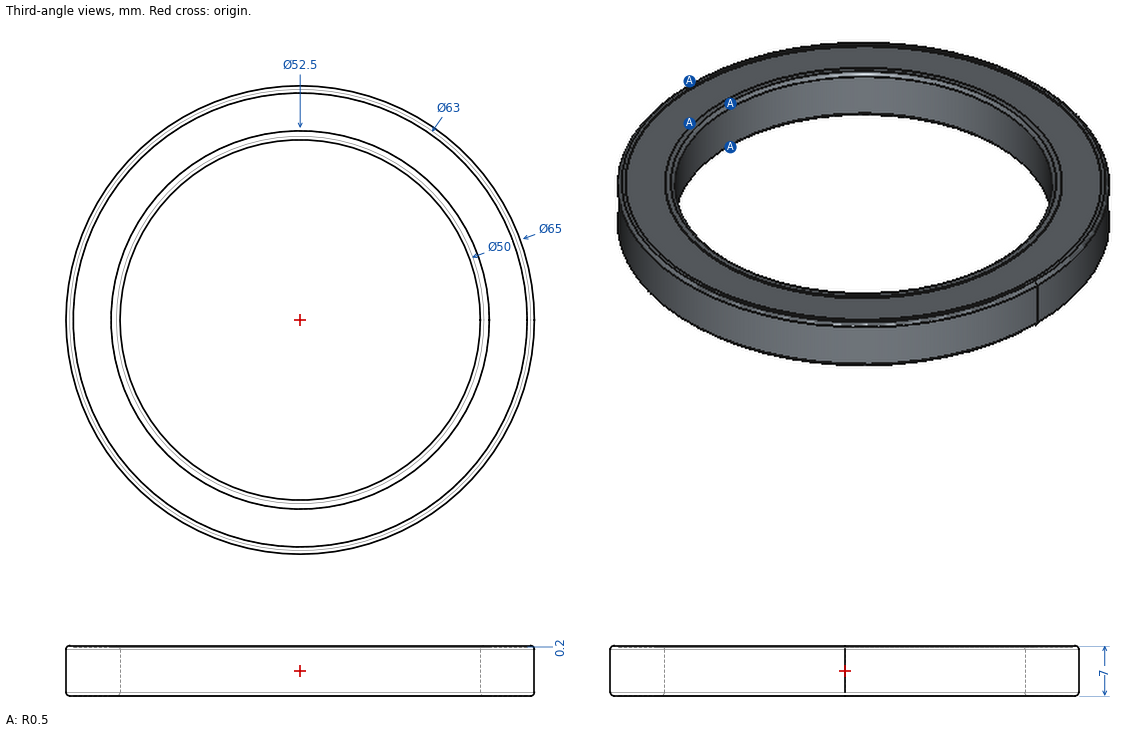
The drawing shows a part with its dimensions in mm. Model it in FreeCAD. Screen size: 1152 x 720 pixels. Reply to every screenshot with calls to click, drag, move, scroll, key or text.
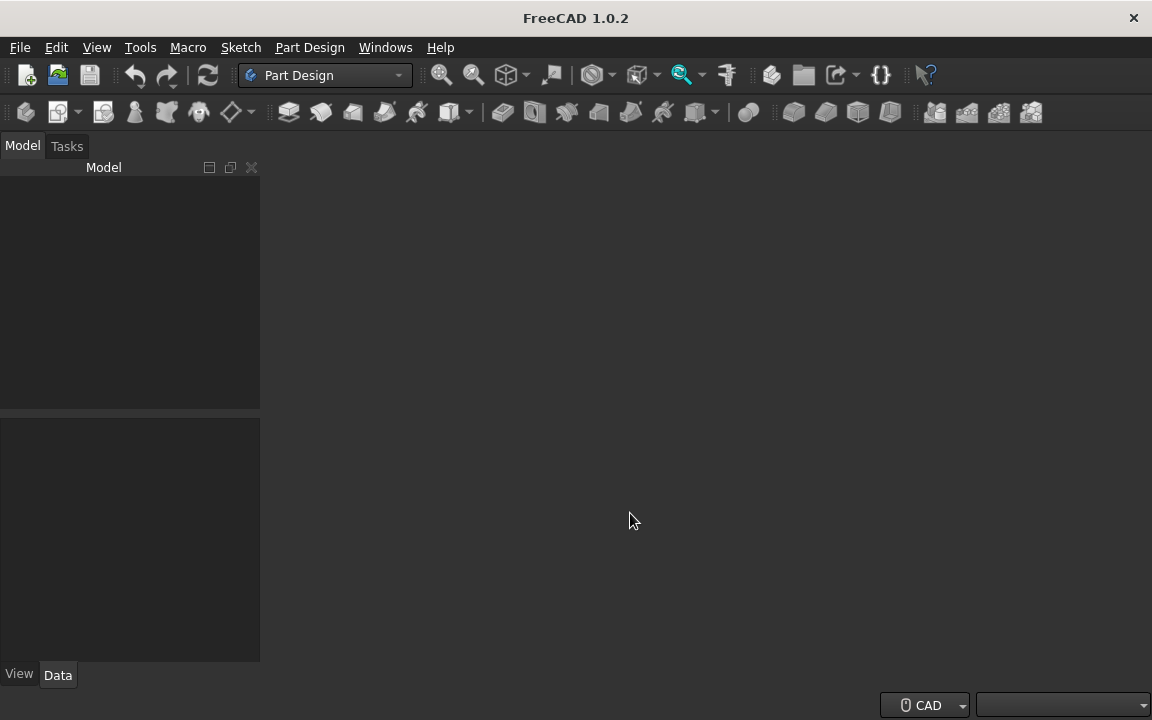
key(ctrl+n)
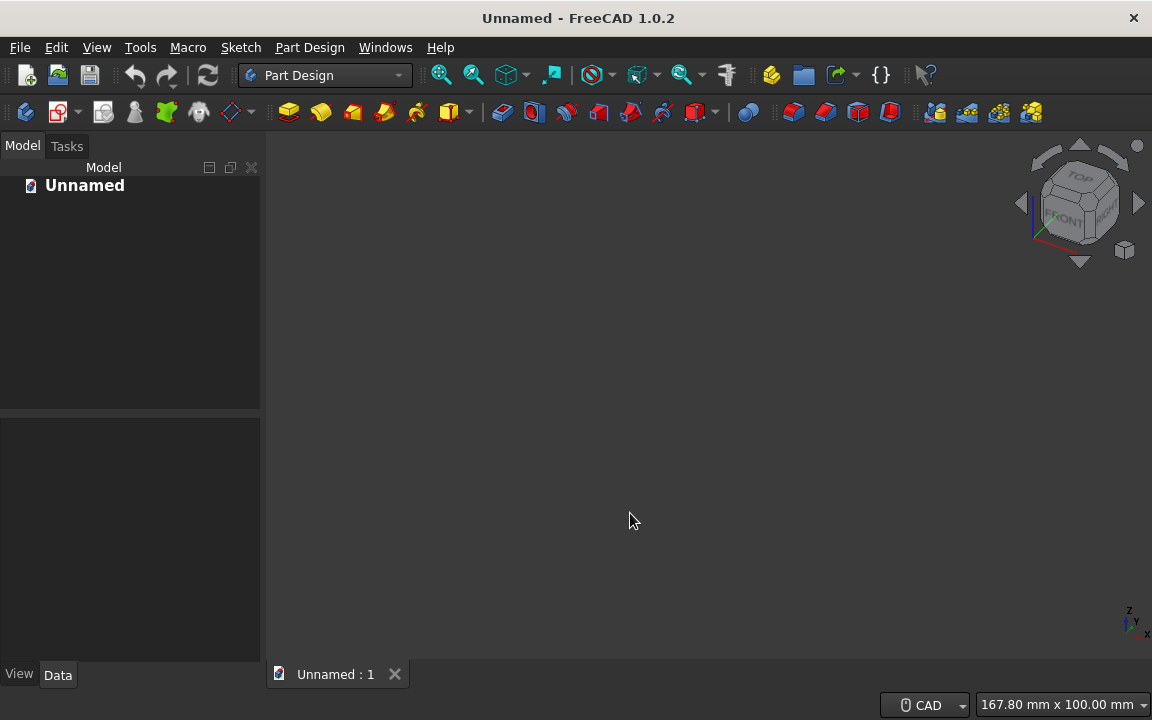
click(58, 112)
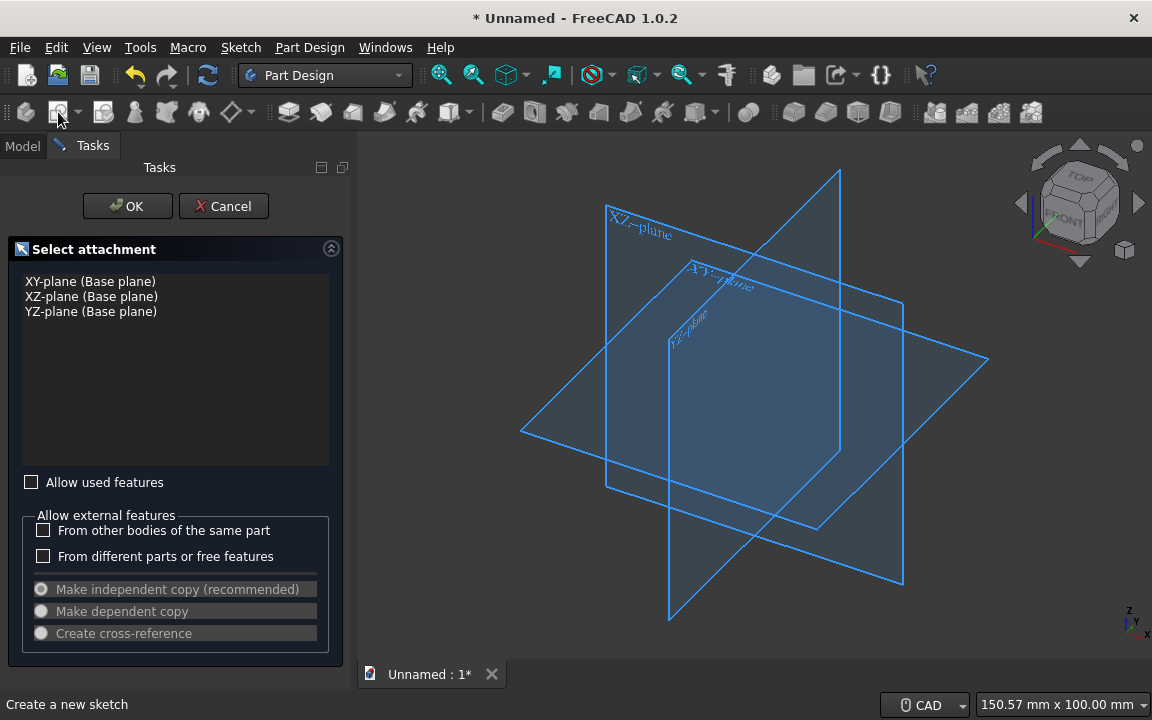
click(82, 282)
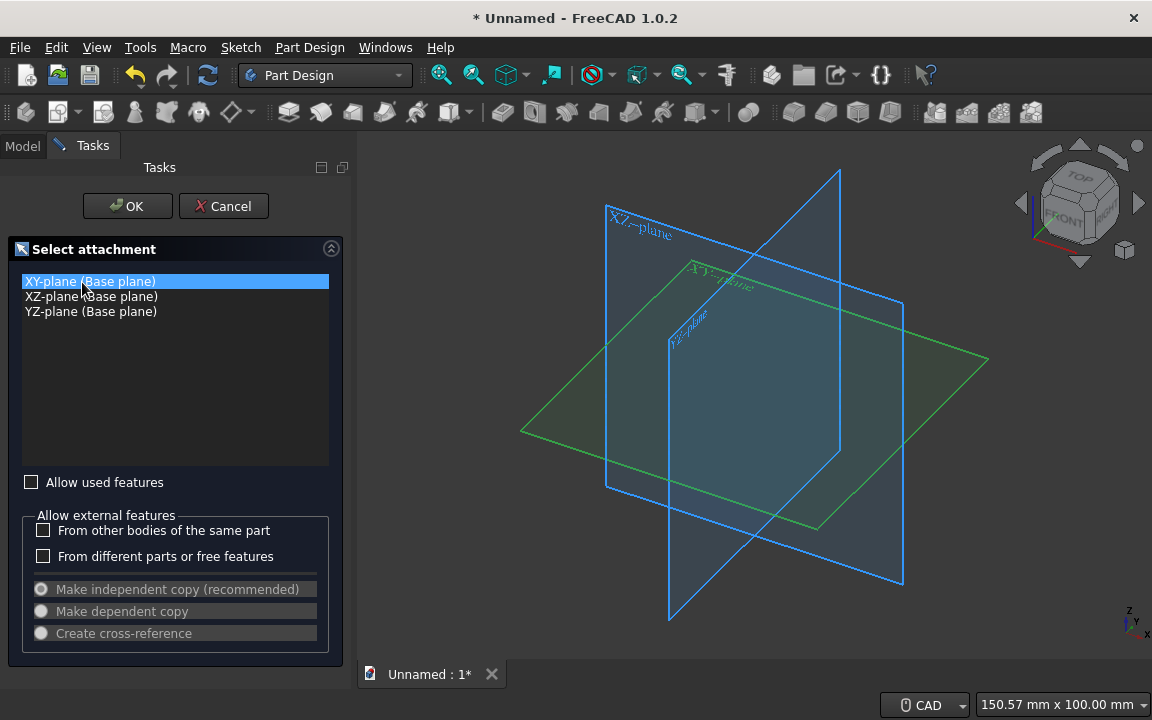
click(128, 206)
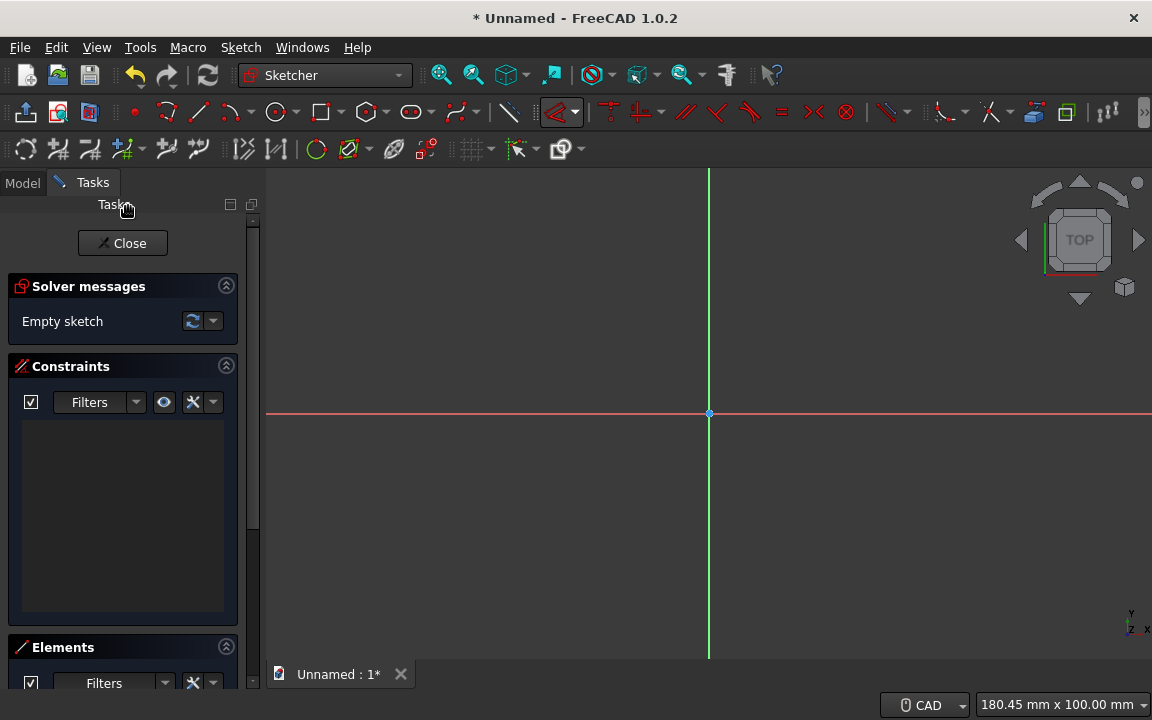
click(276, 112)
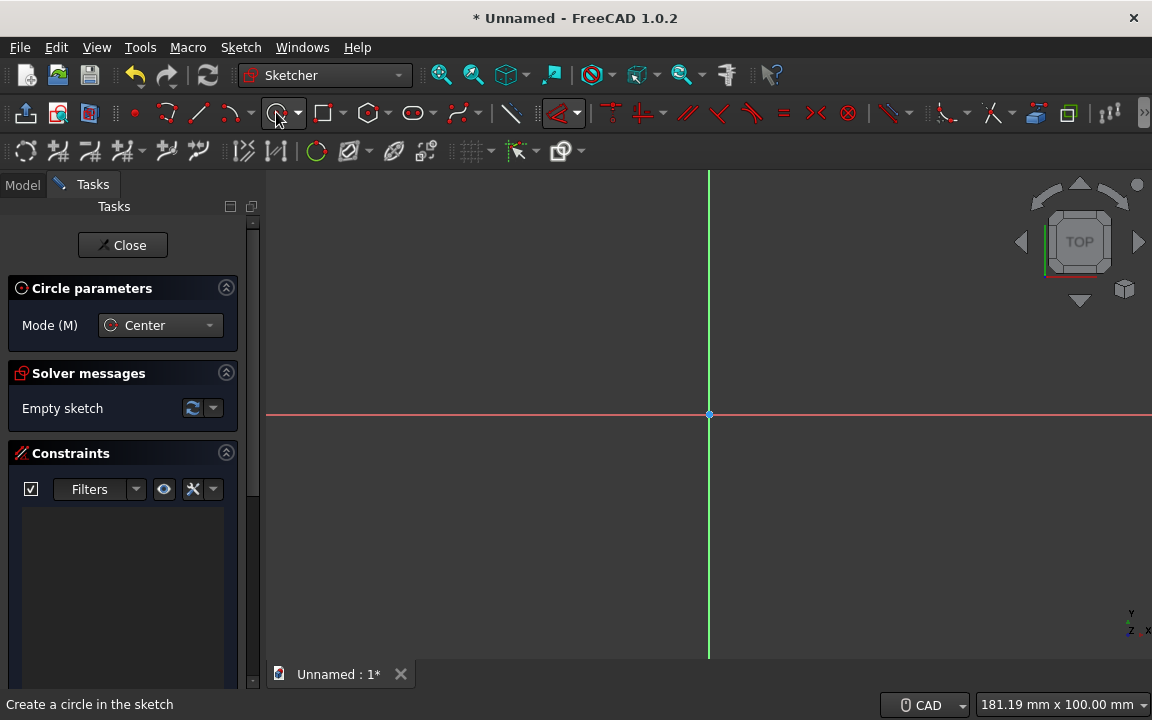
click(709, 414)
click(821, 302)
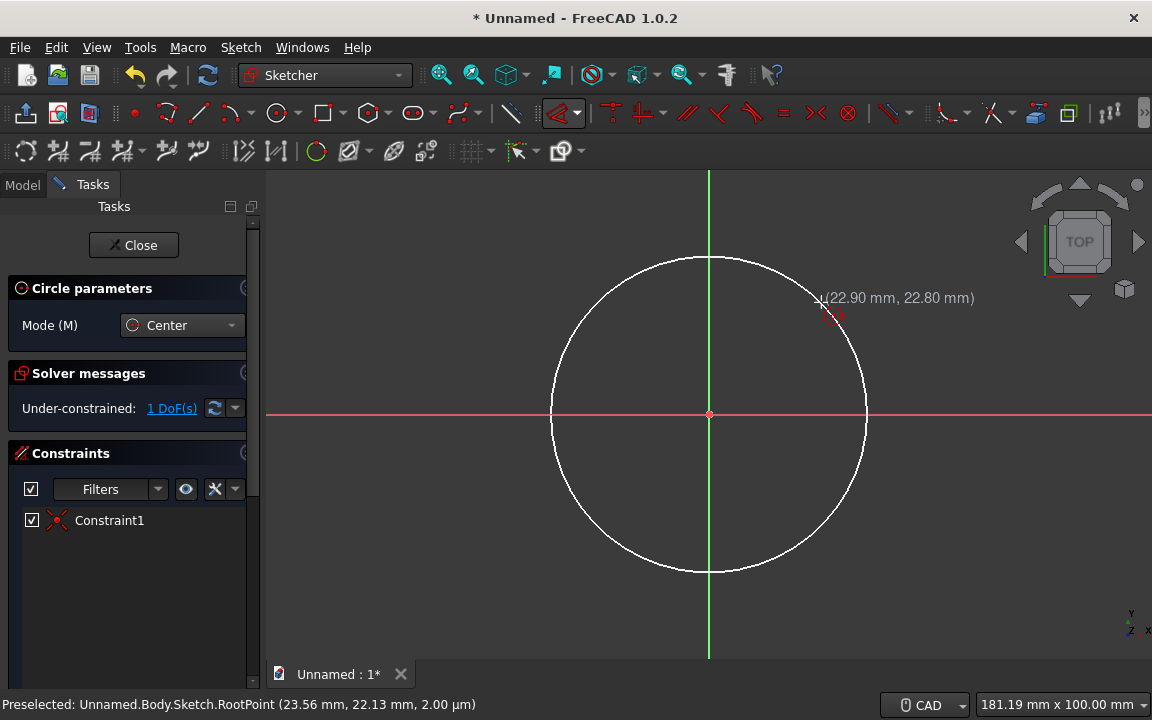
click(709, 414)
click(795, 328)
key(Escape)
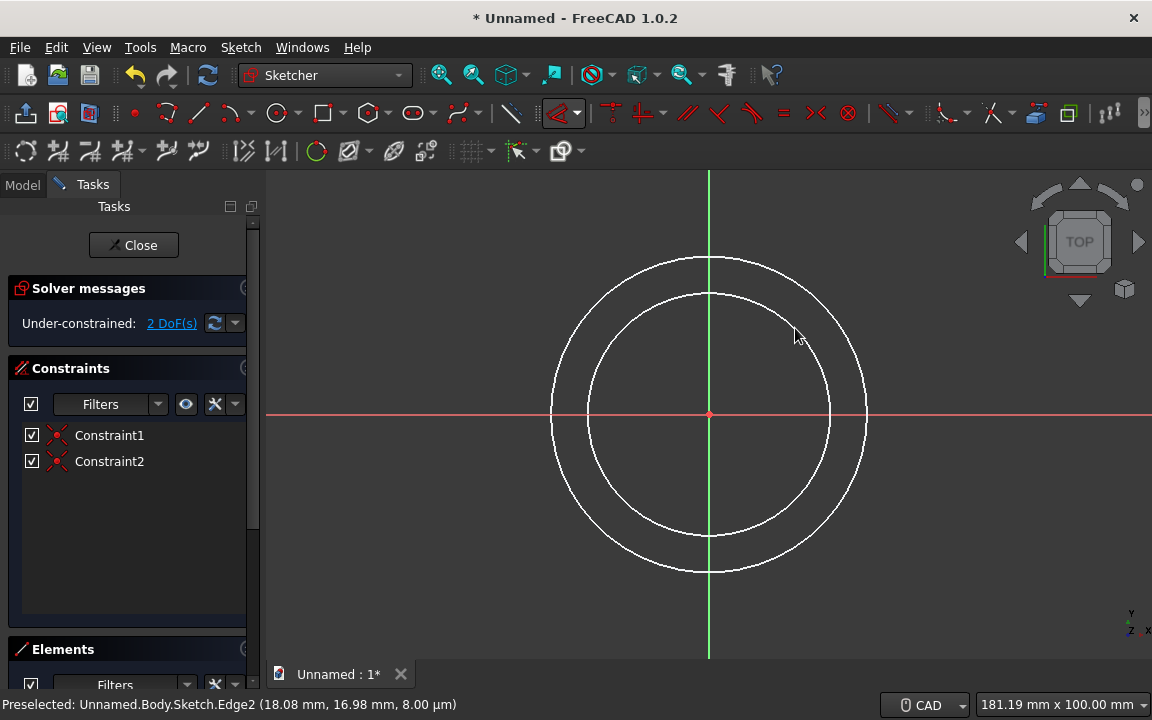
click(820, 302)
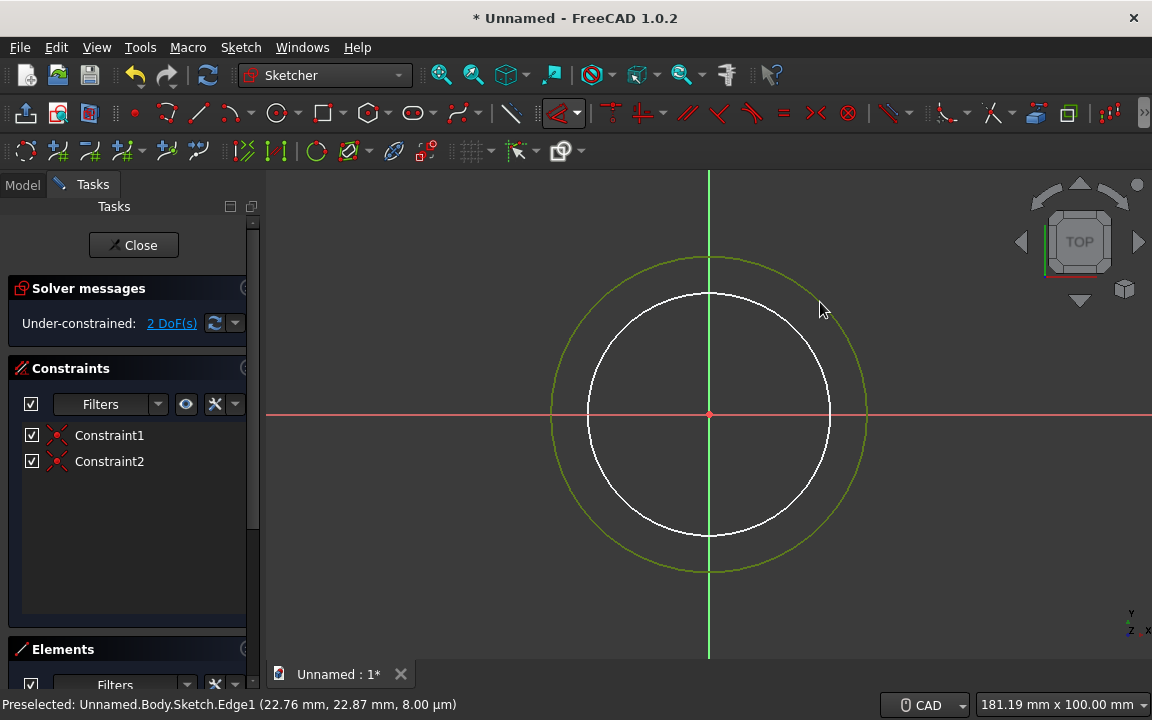
click(580, 114)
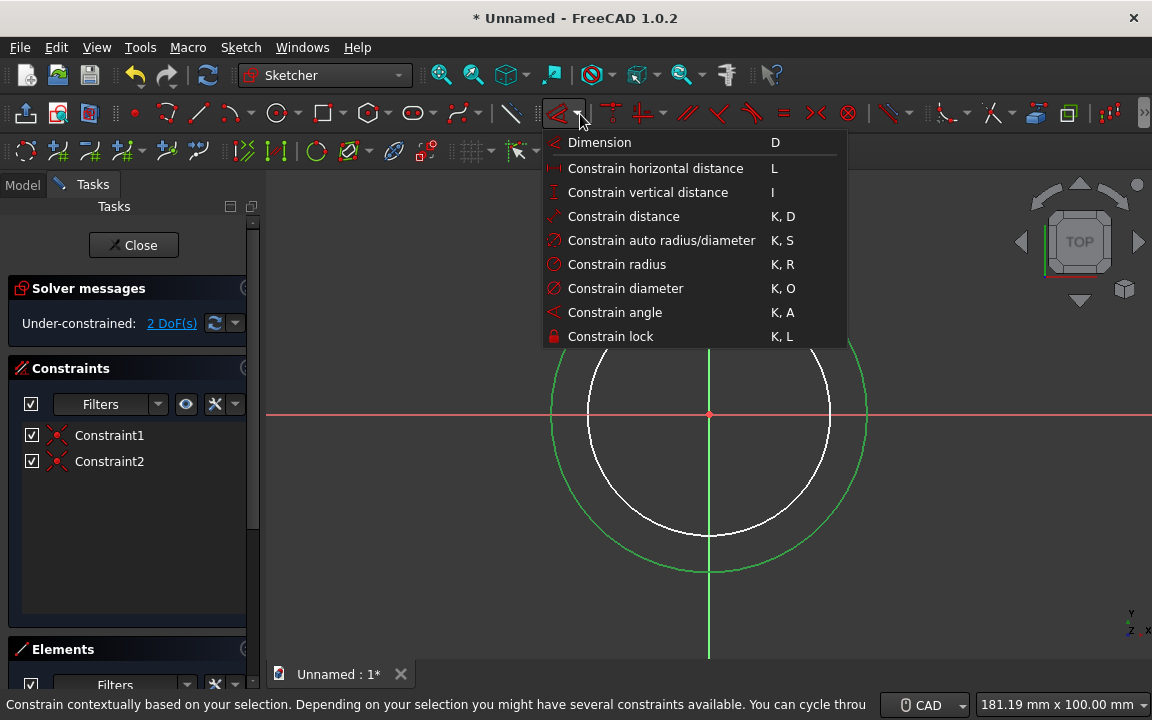
click(695, 288)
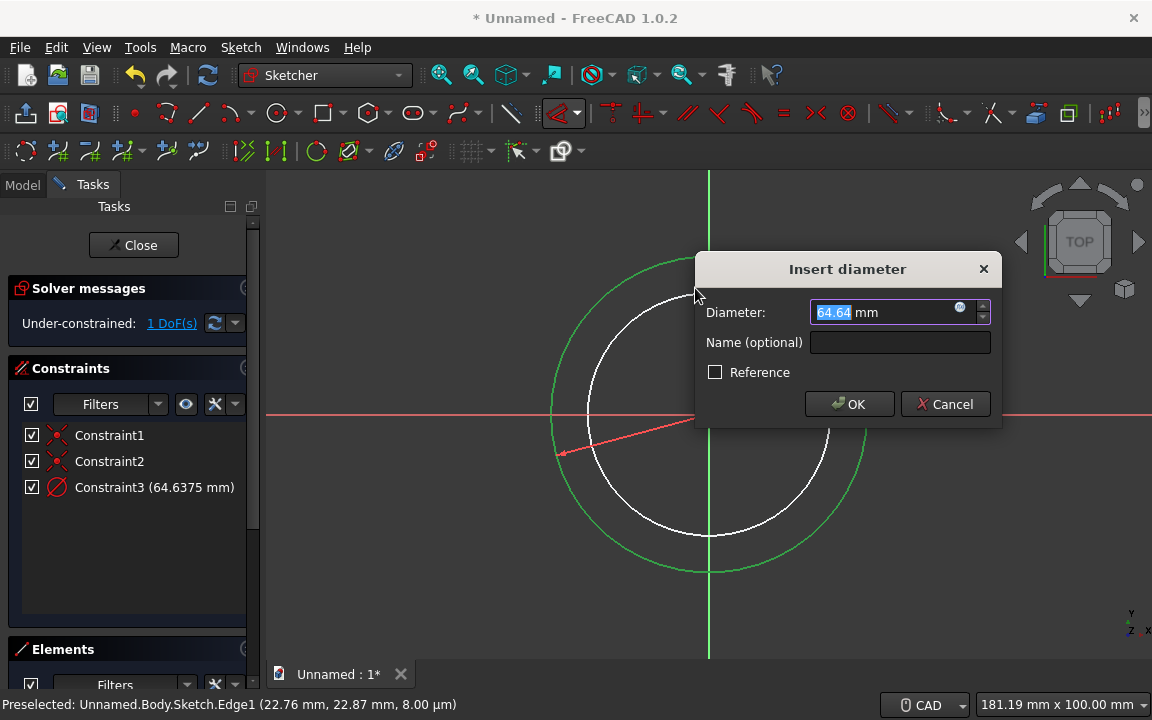
text(65)
key(Return)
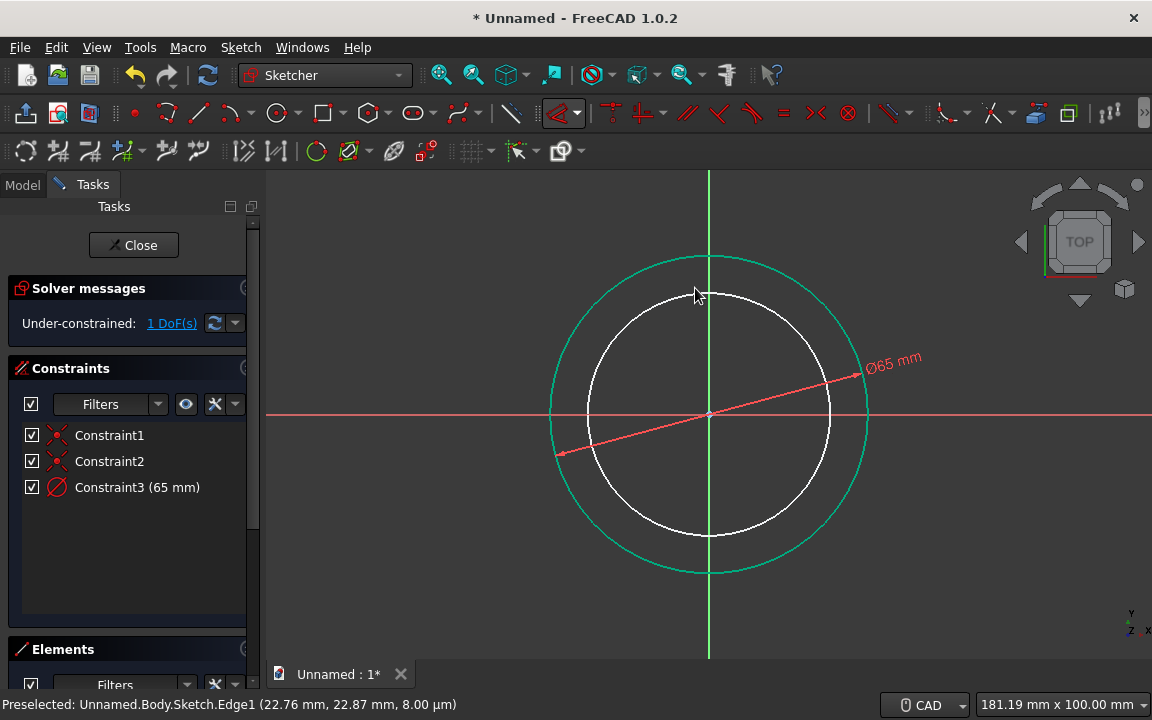
click(794, 328)